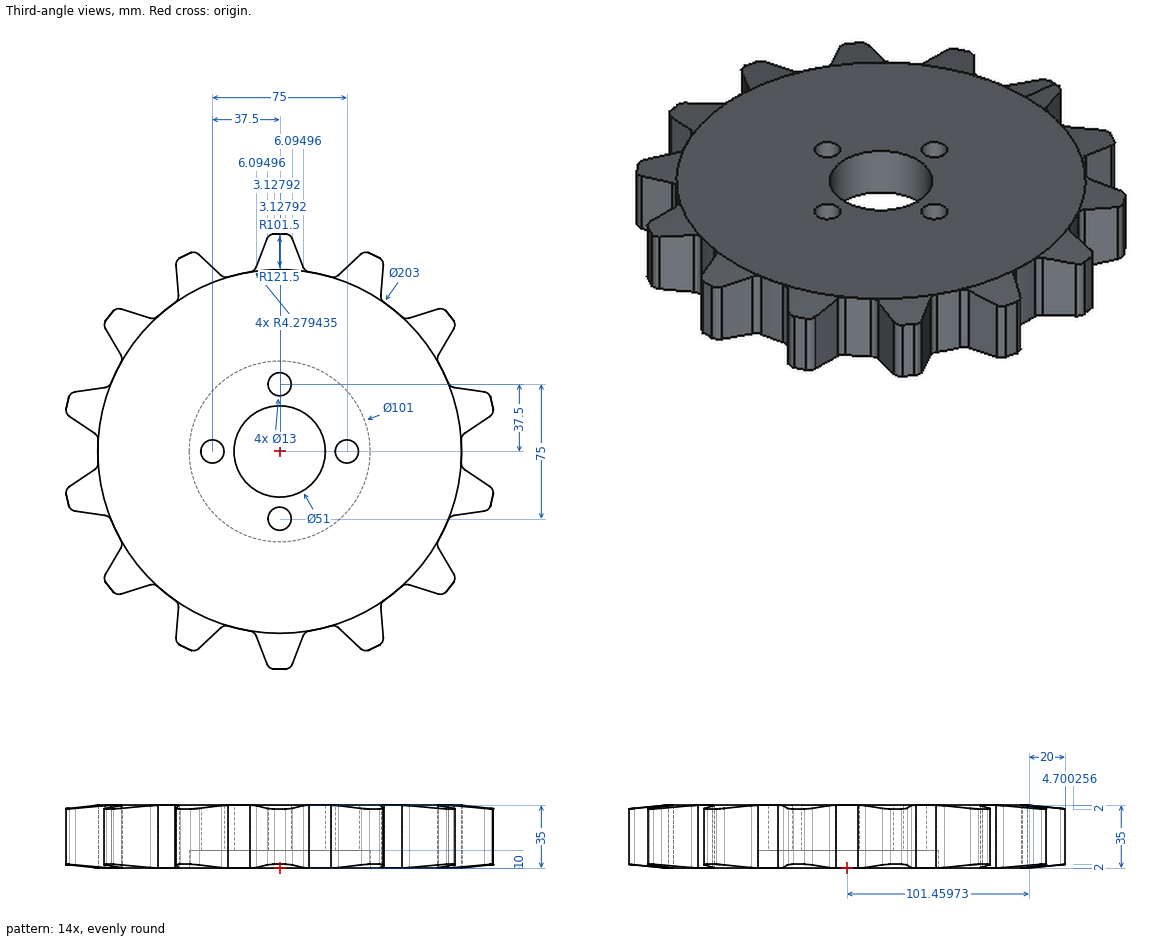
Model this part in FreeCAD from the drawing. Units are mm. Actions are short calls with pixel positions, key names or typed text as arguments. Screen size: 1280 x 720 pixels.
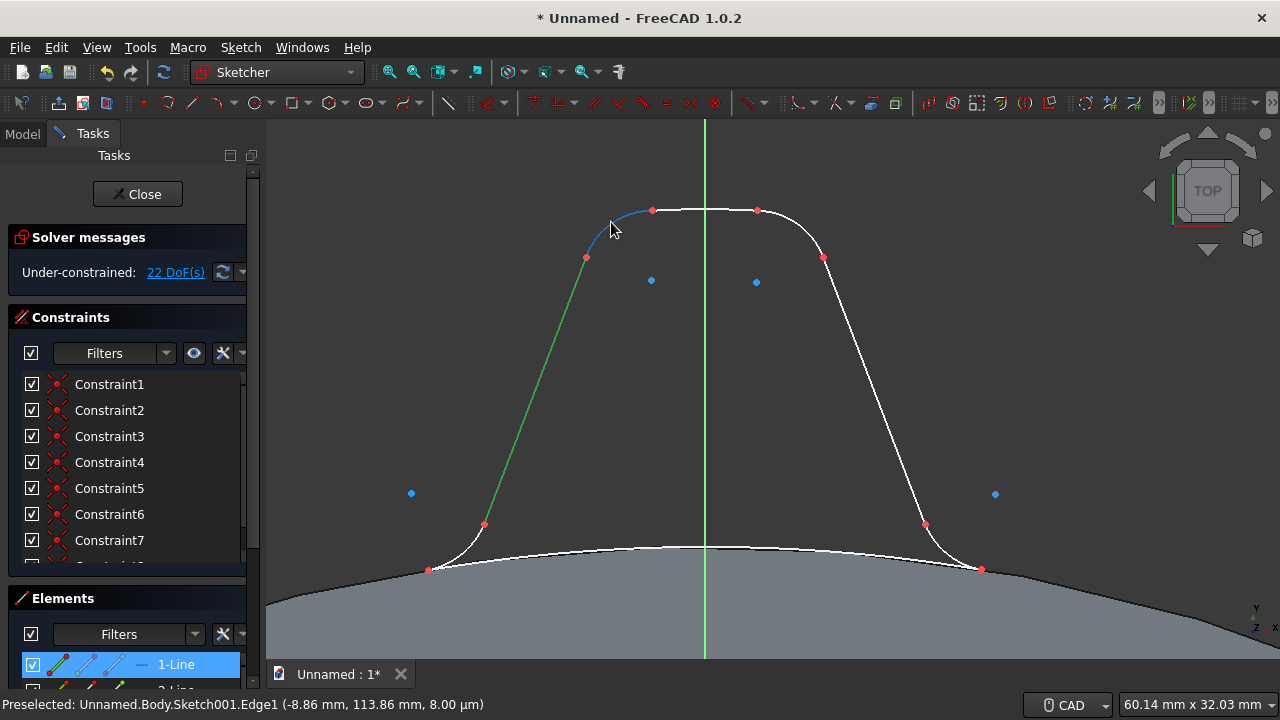
click(472, 544)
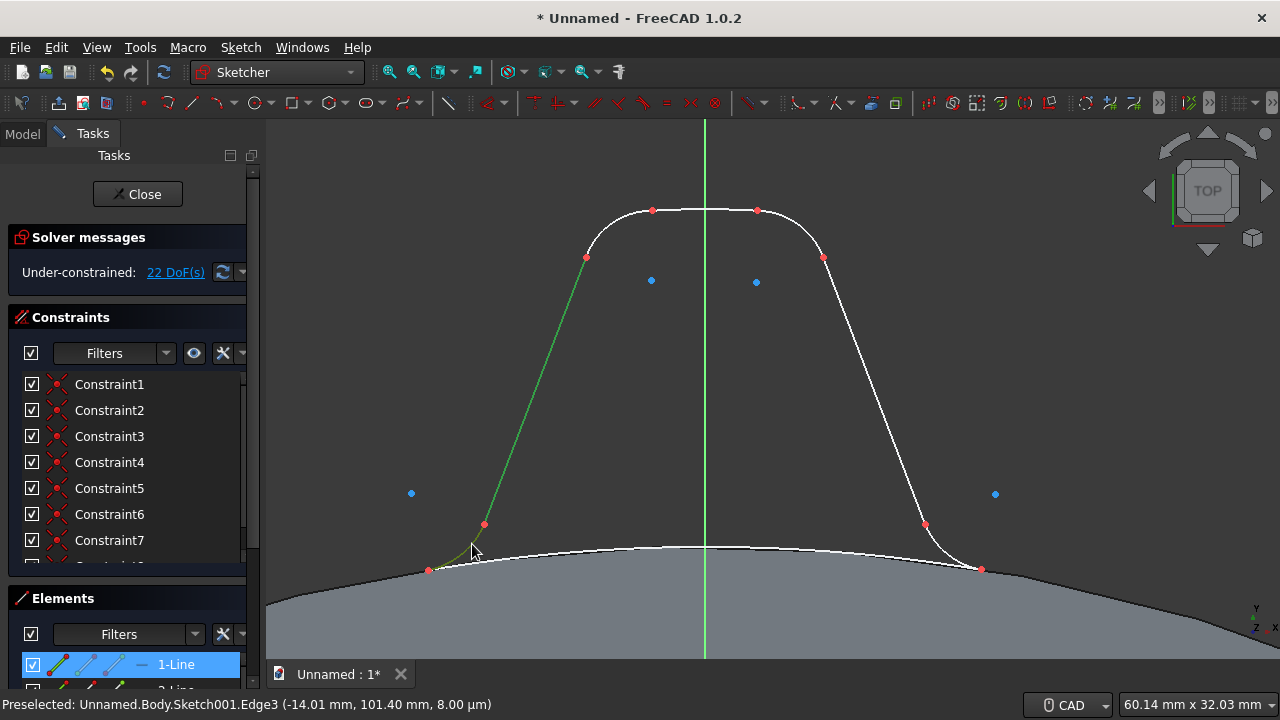
click(644, 104)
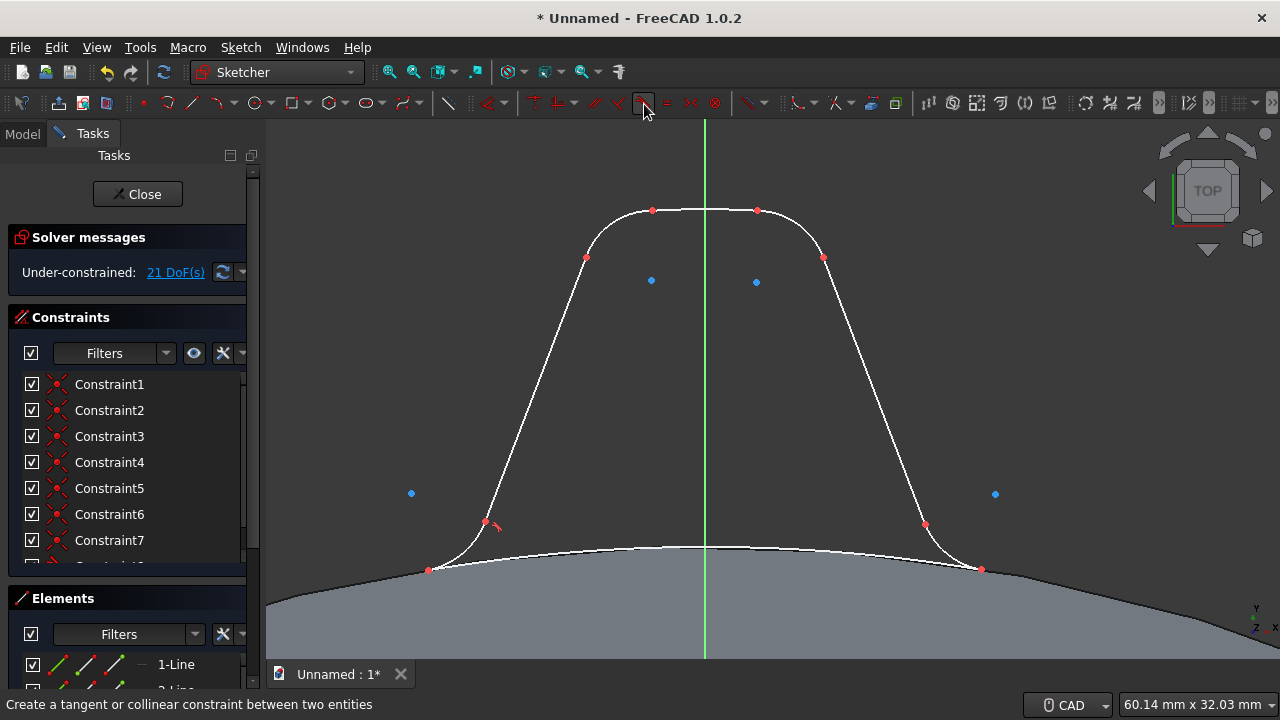
click(556, 337)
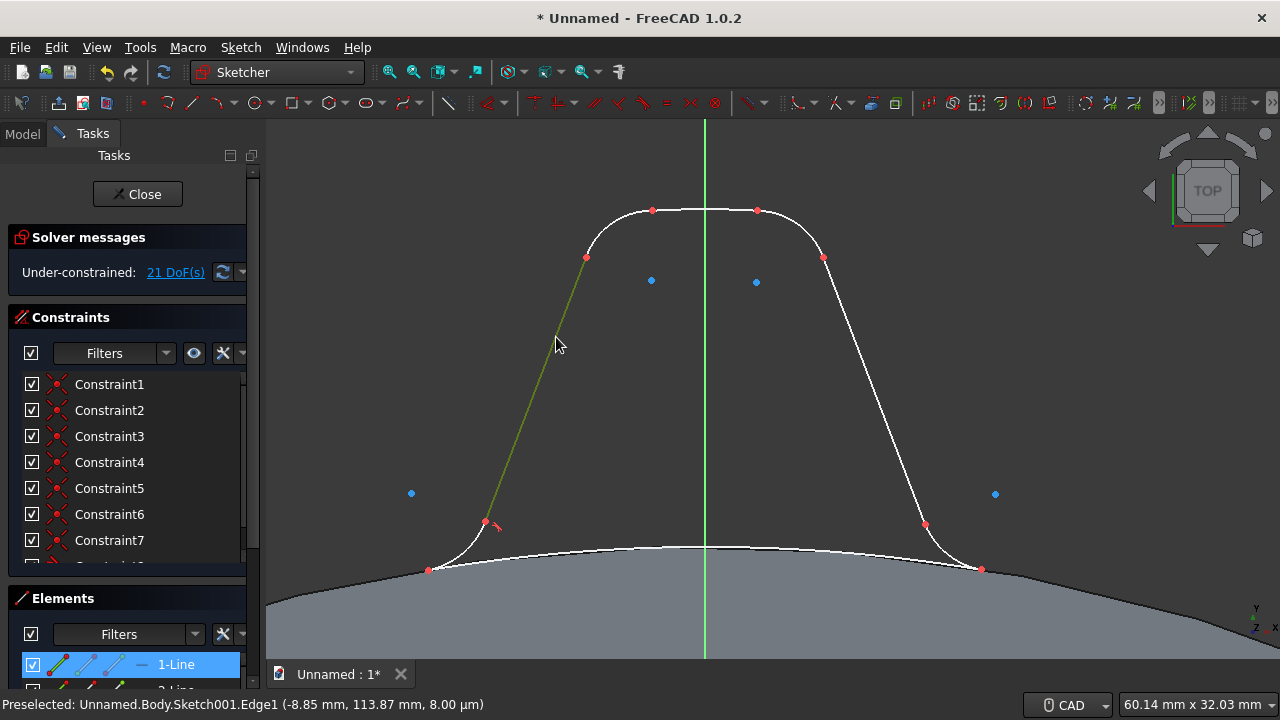
click(627, 215)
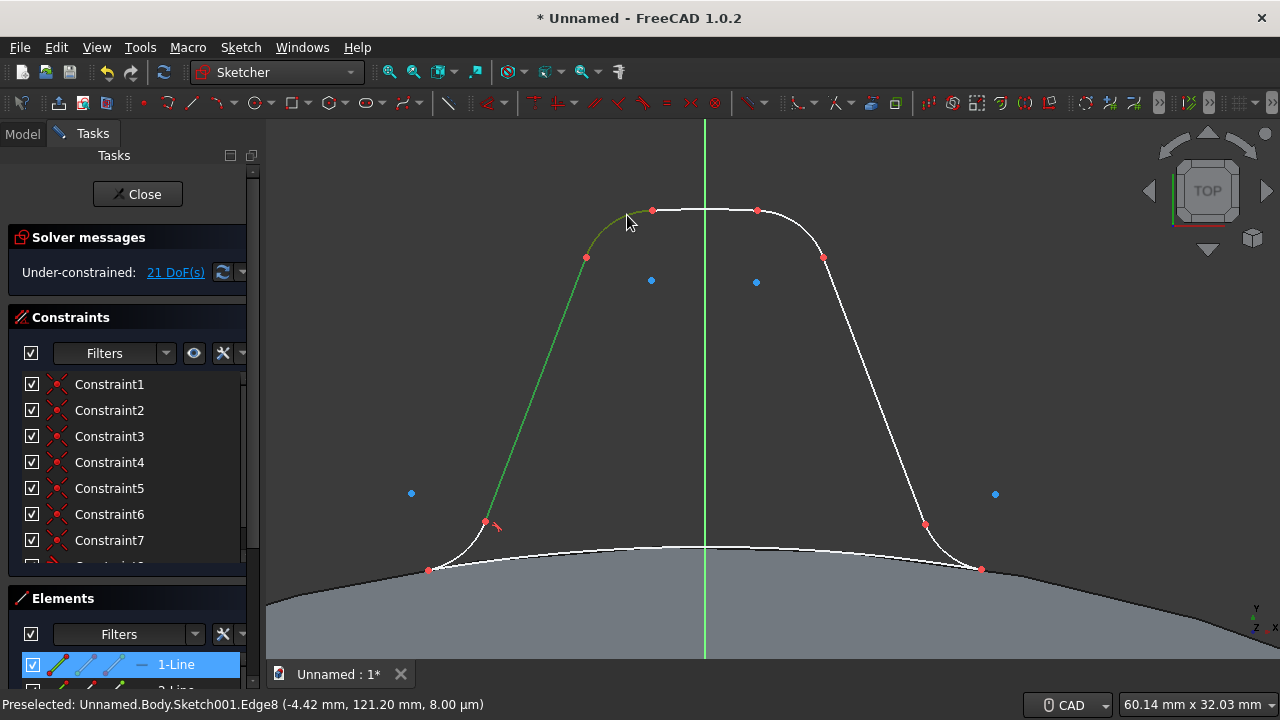
click(644, 104)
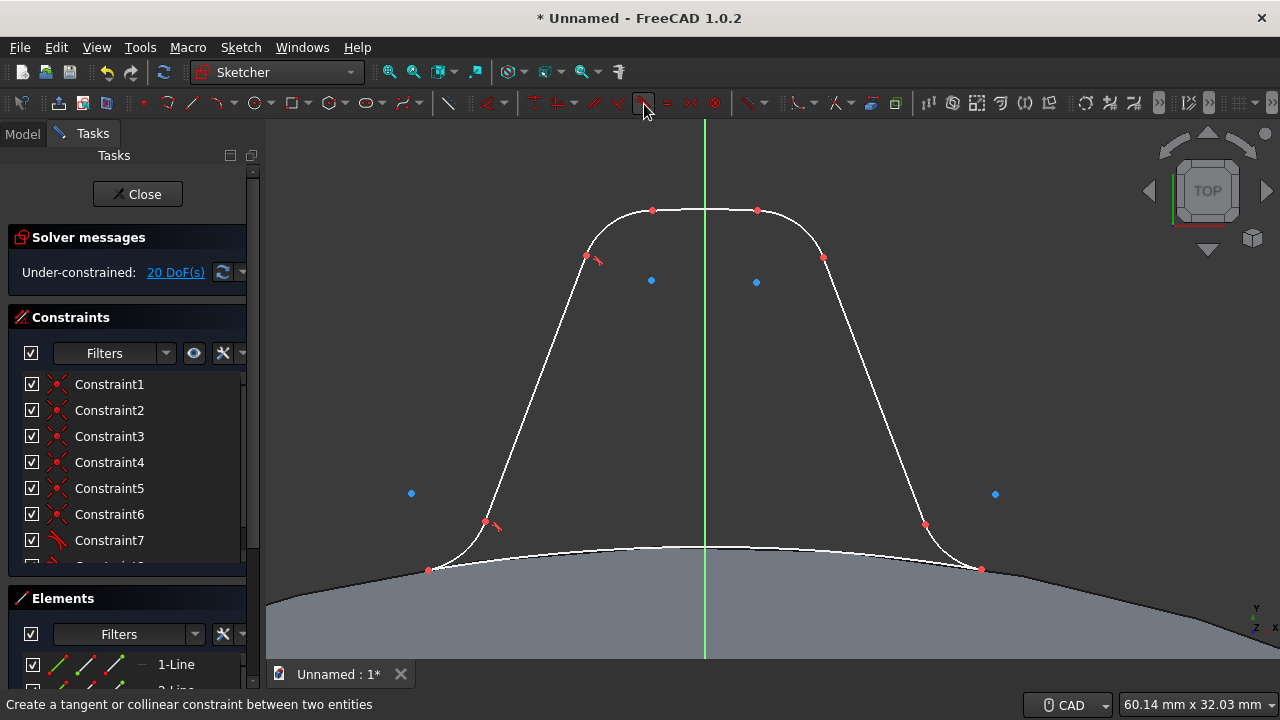
click(894, 444)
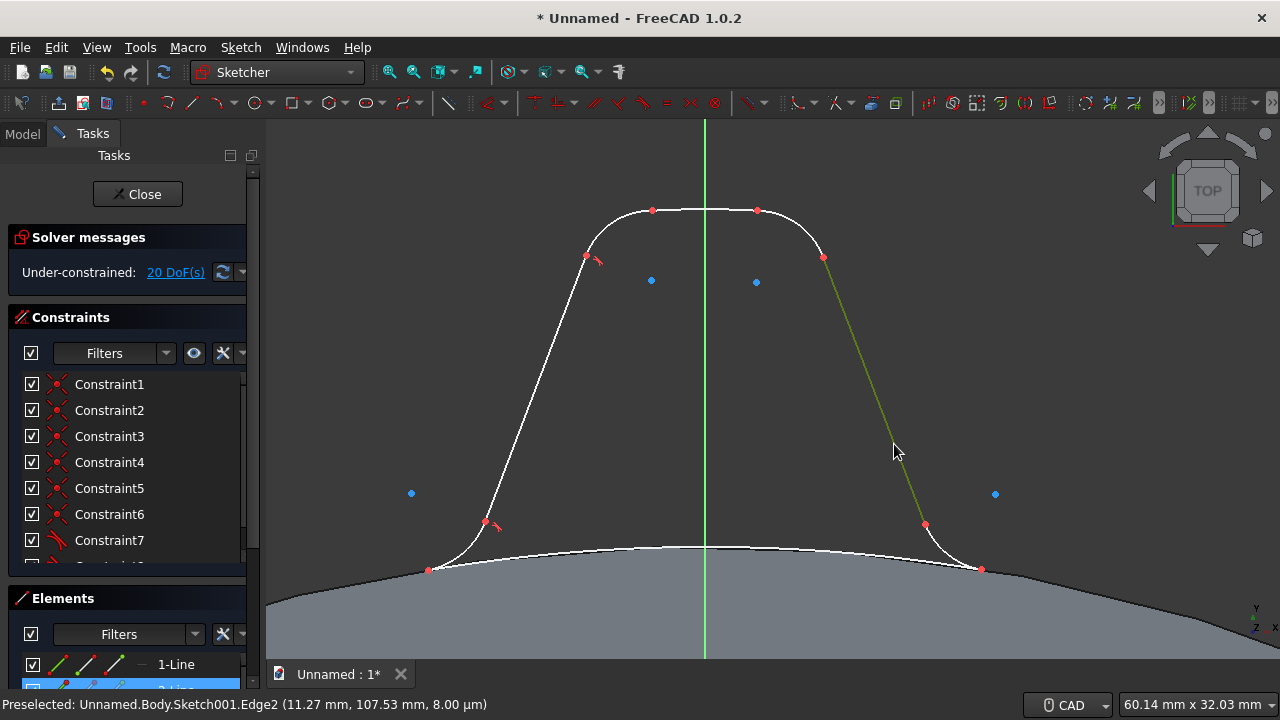
click(937, 544)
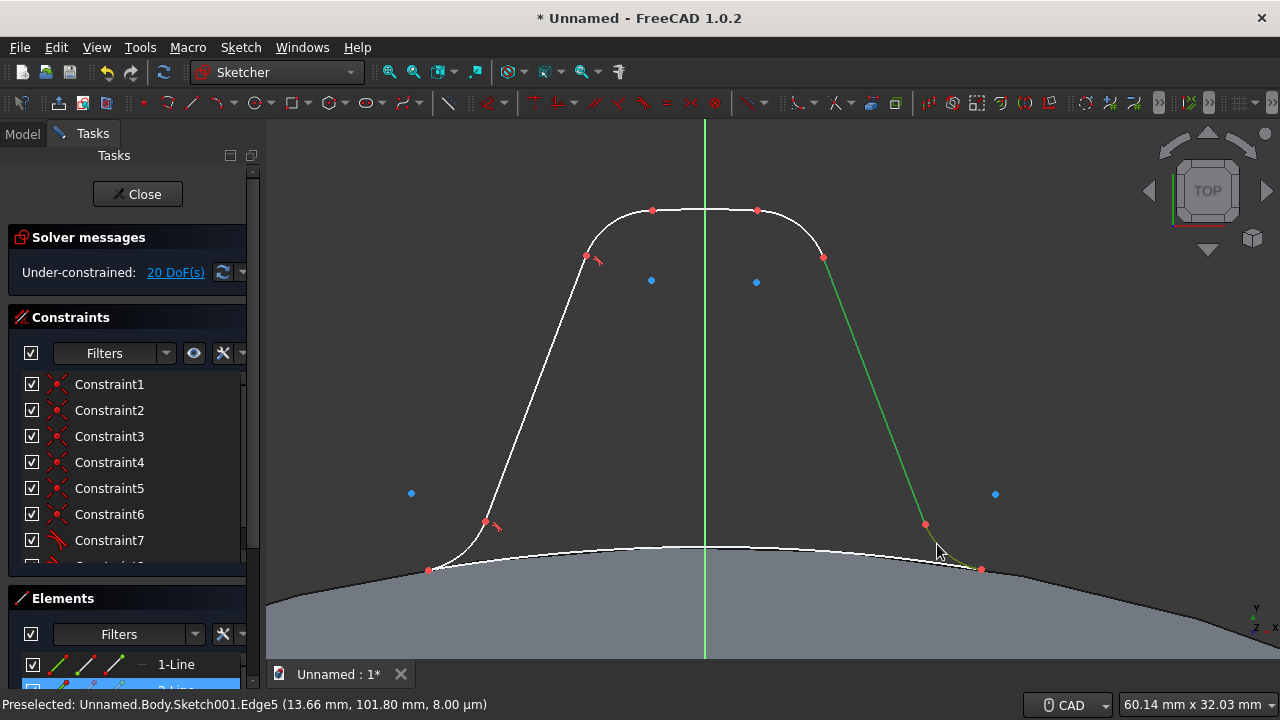
click(644, 104)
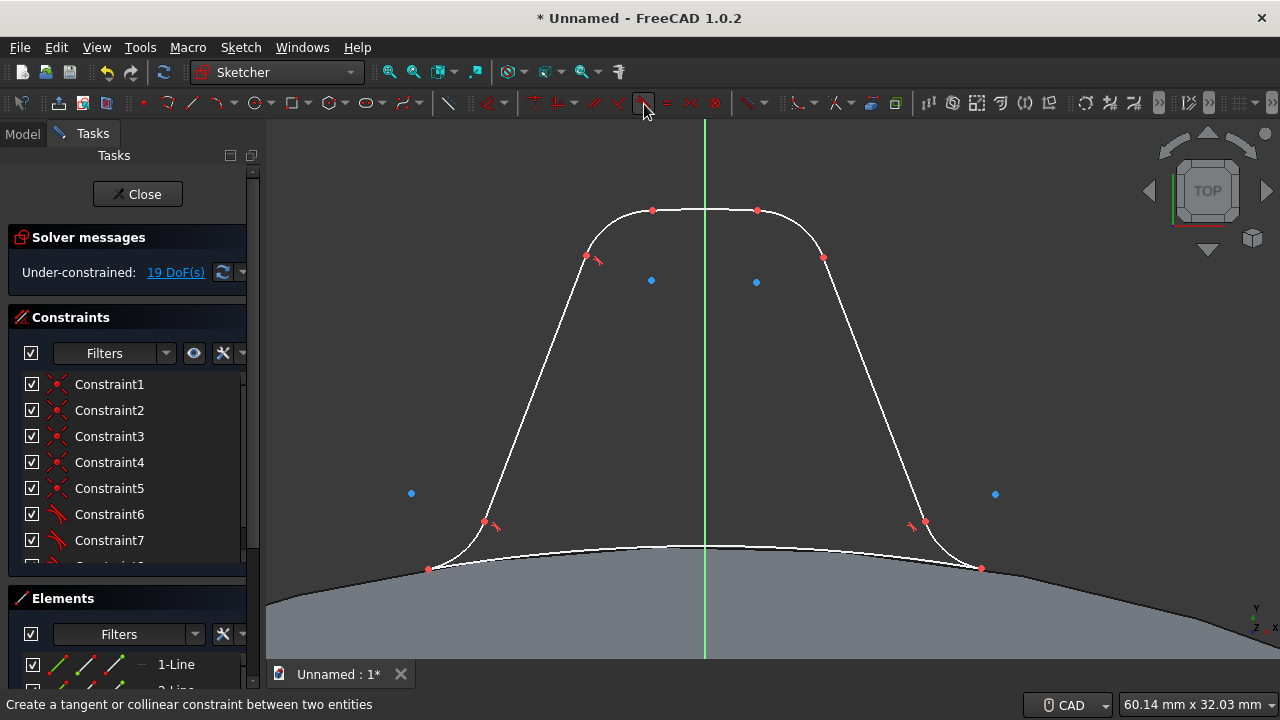
click(894, 443)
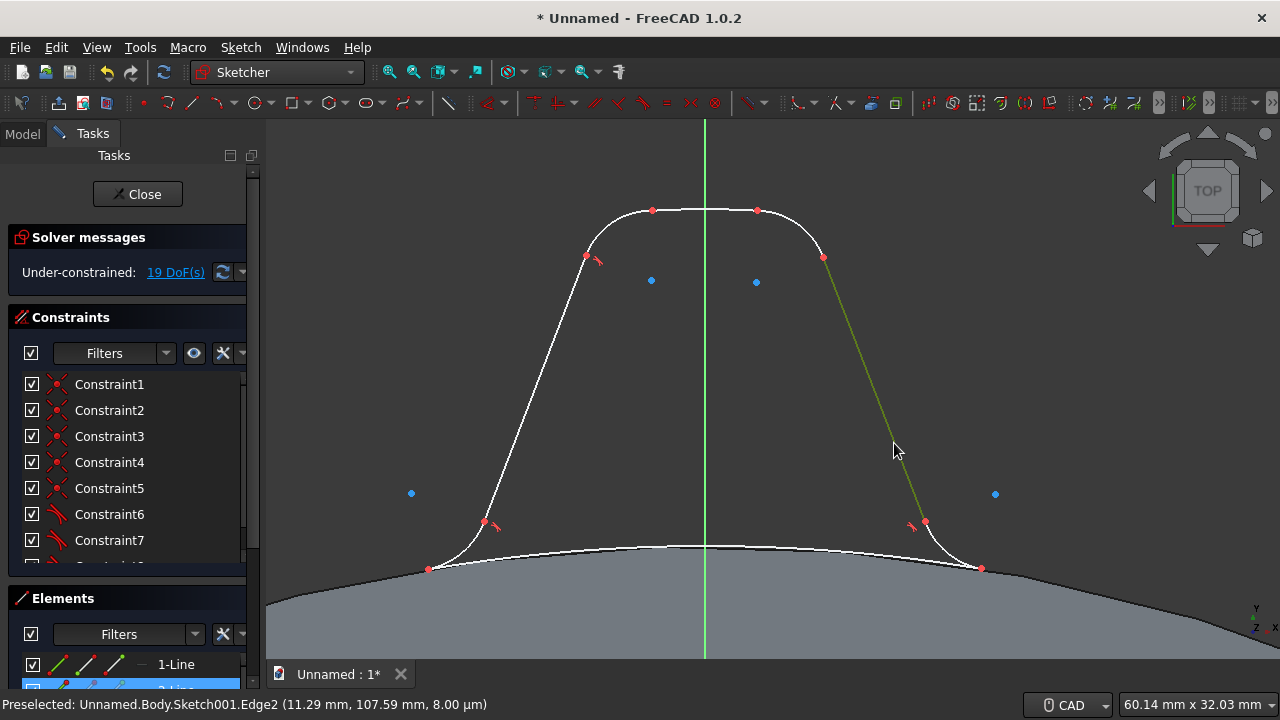
click(810, 235)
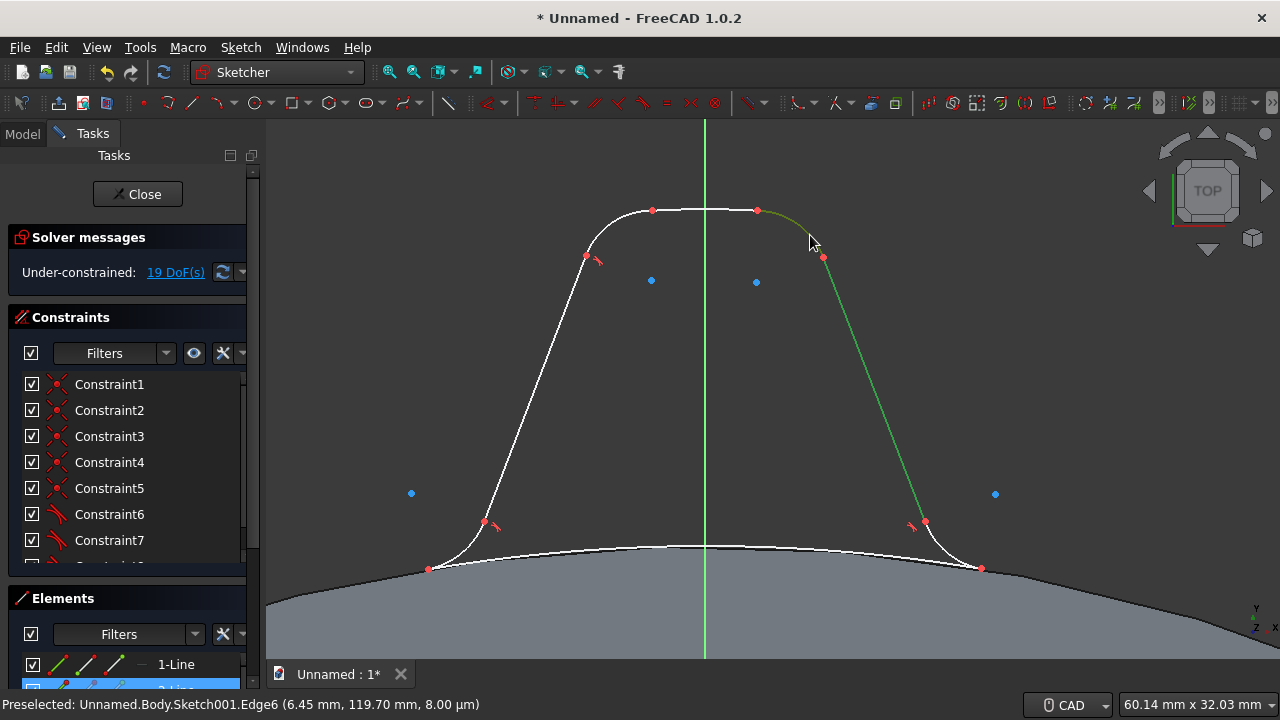
click(644, 104)